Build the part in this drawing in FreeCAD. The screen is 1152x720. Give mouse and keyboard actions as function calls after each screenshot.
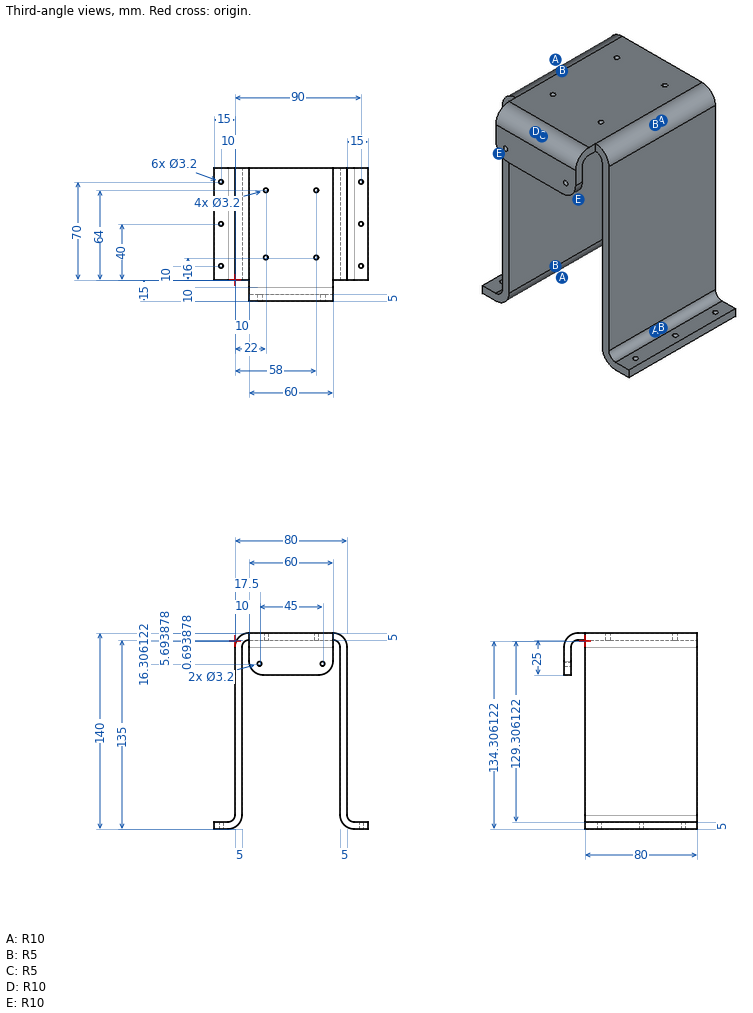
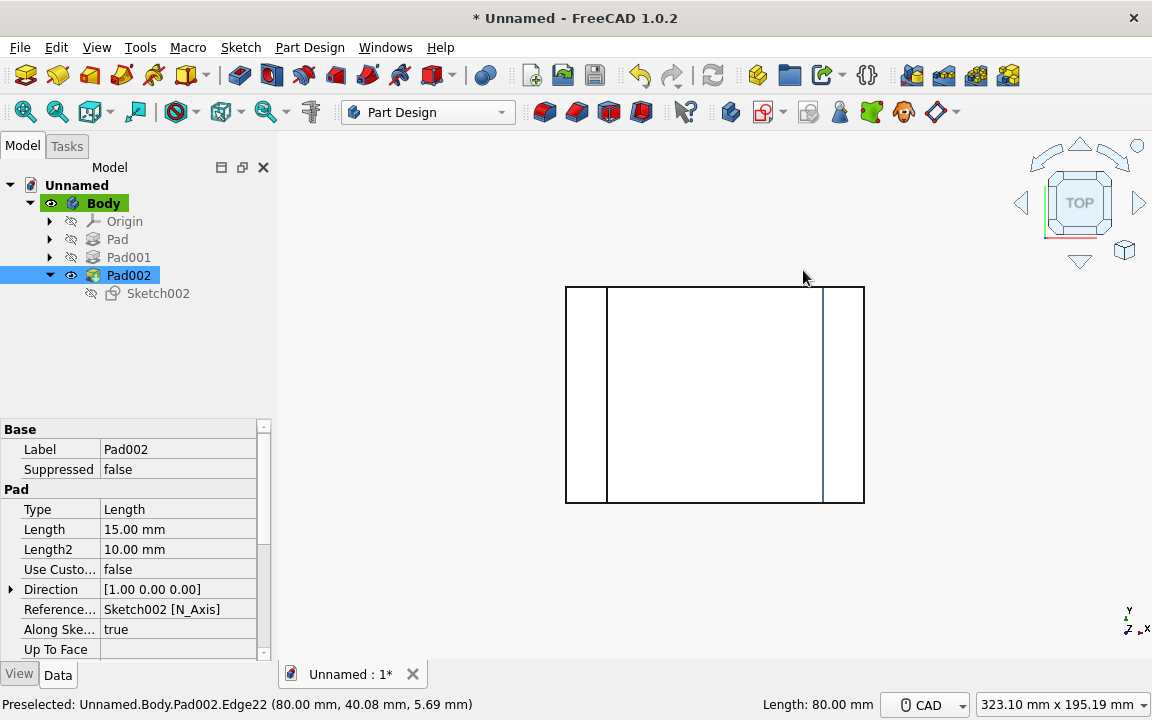
click(26, 112)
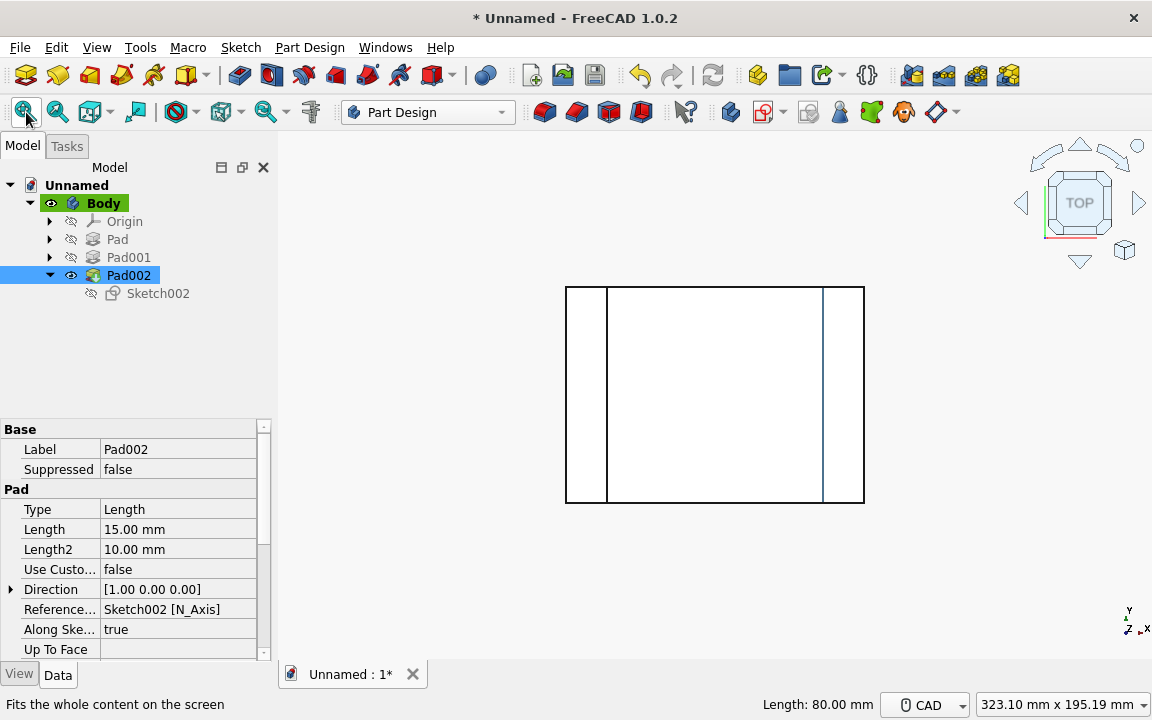
click(607, 394, ctrl)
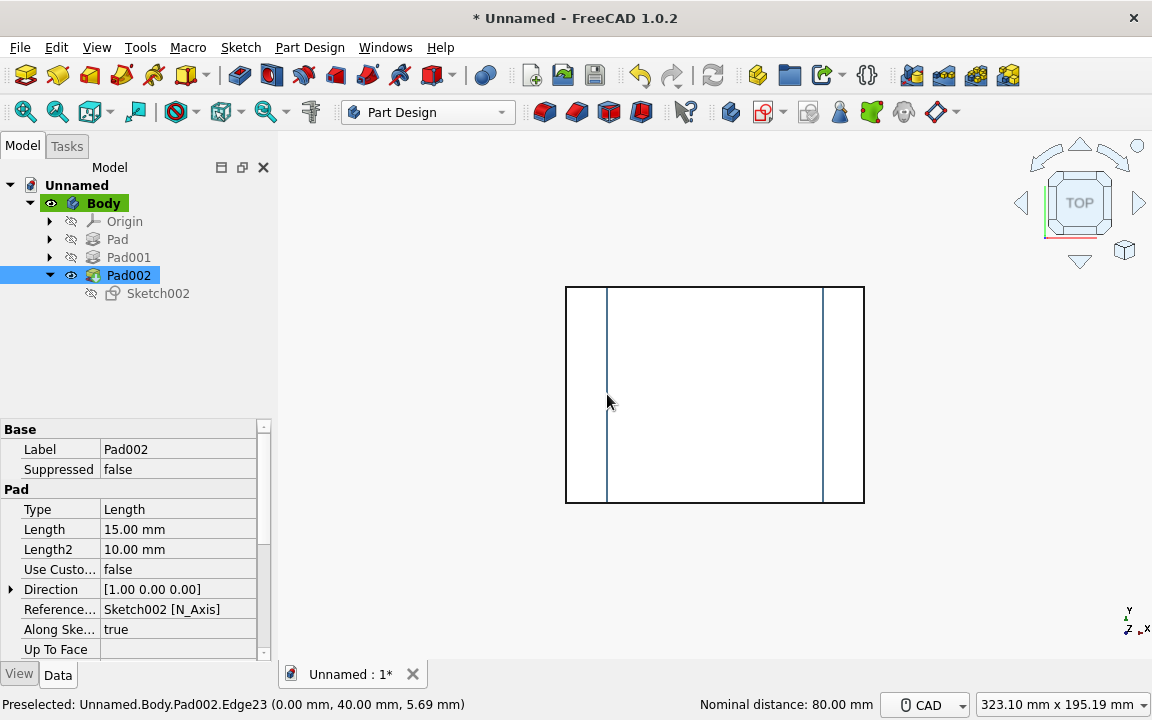
key(1)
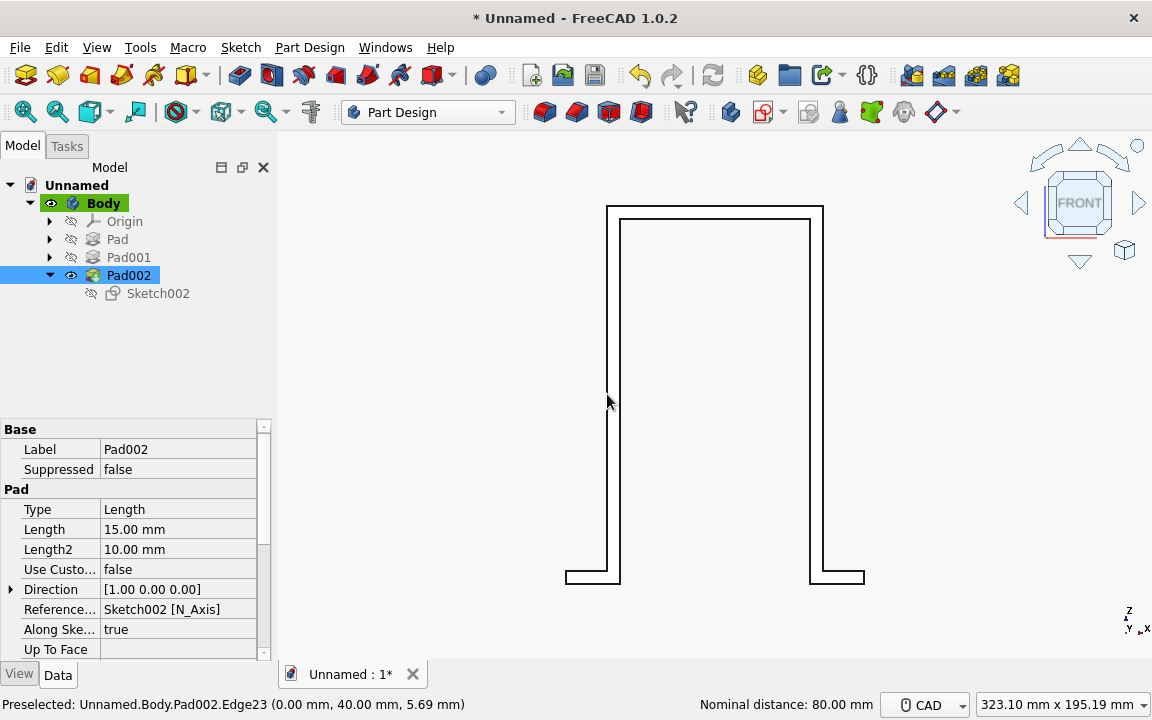
key(3)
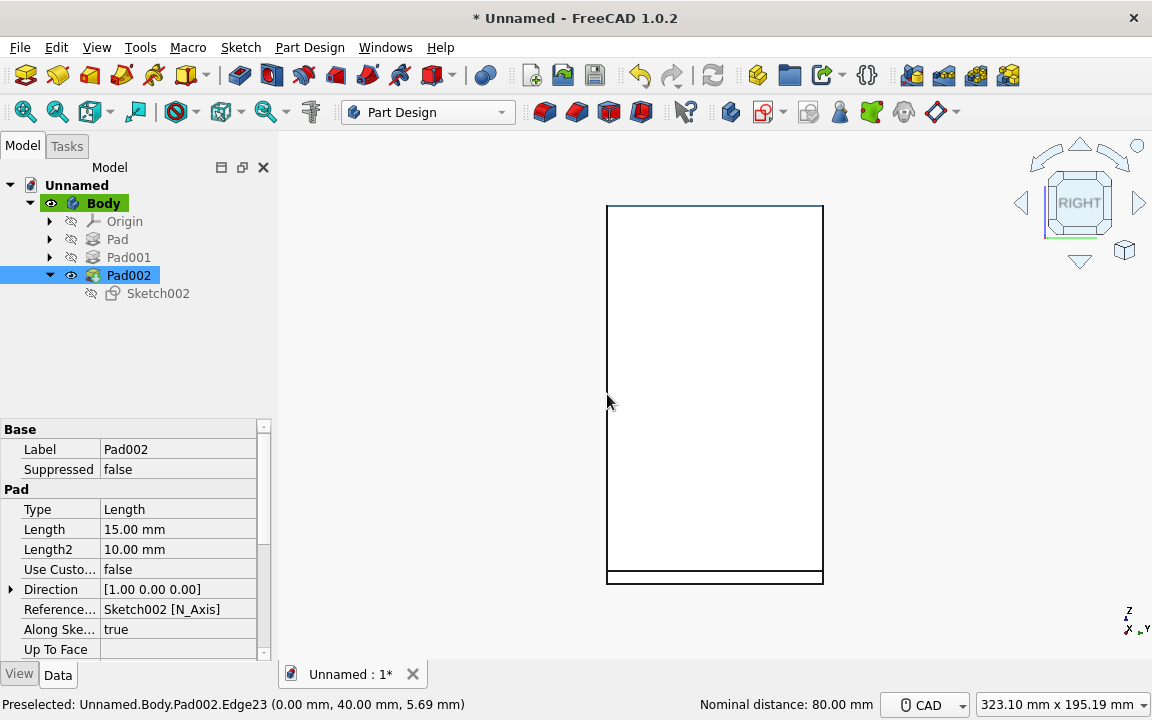
key(5)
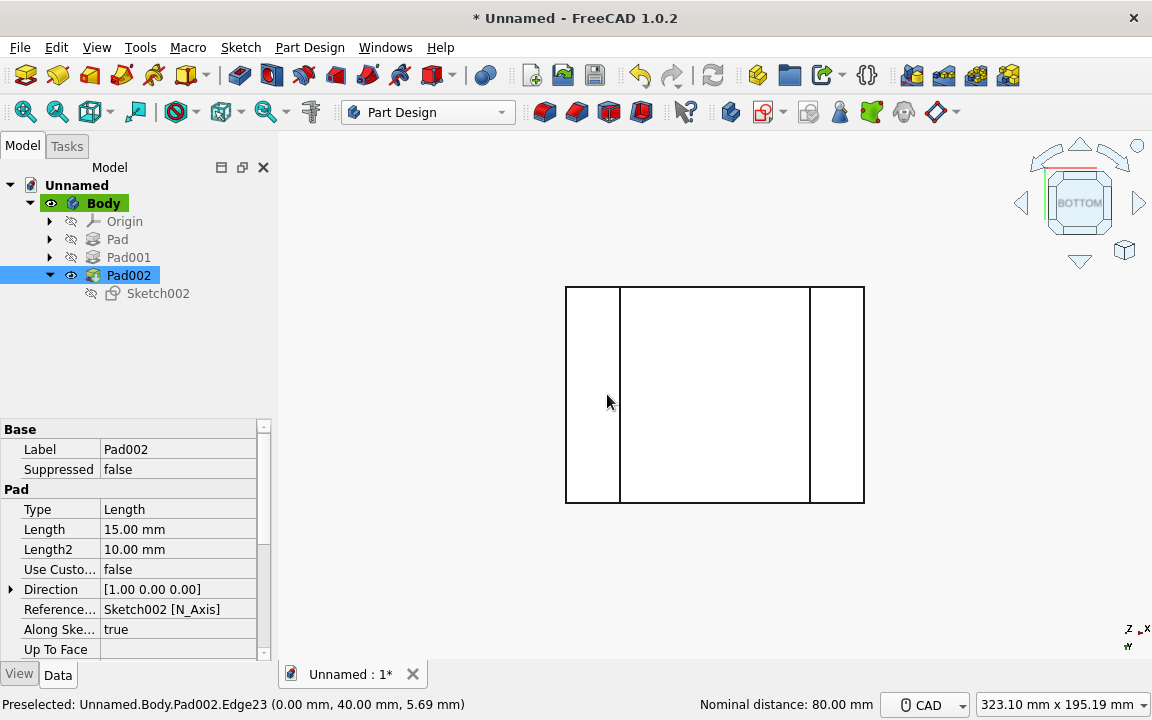
click(26, 112)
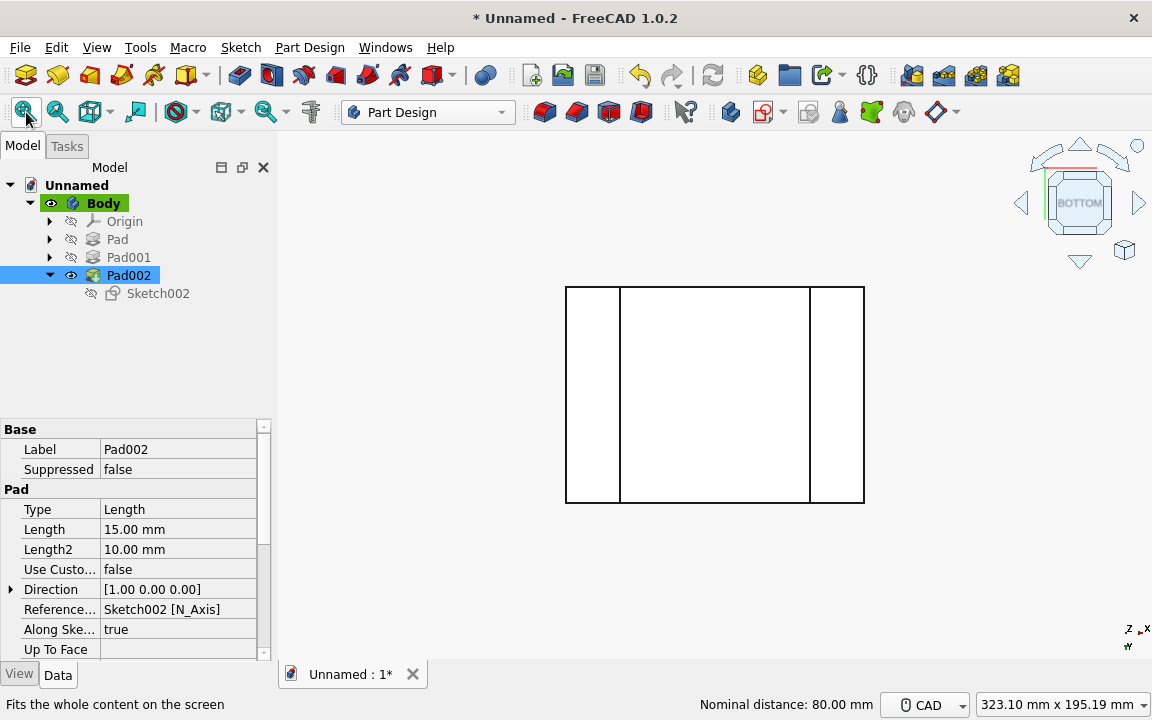
click(620, 394, ctrl)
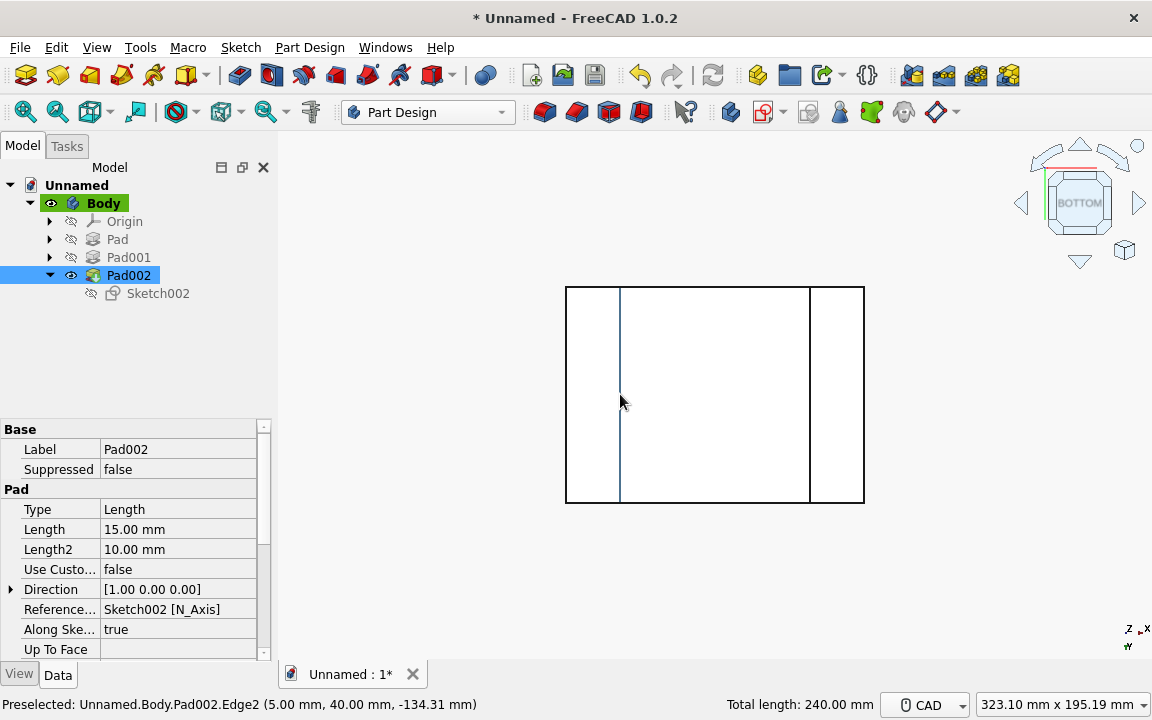
click(810, 394, ctrl)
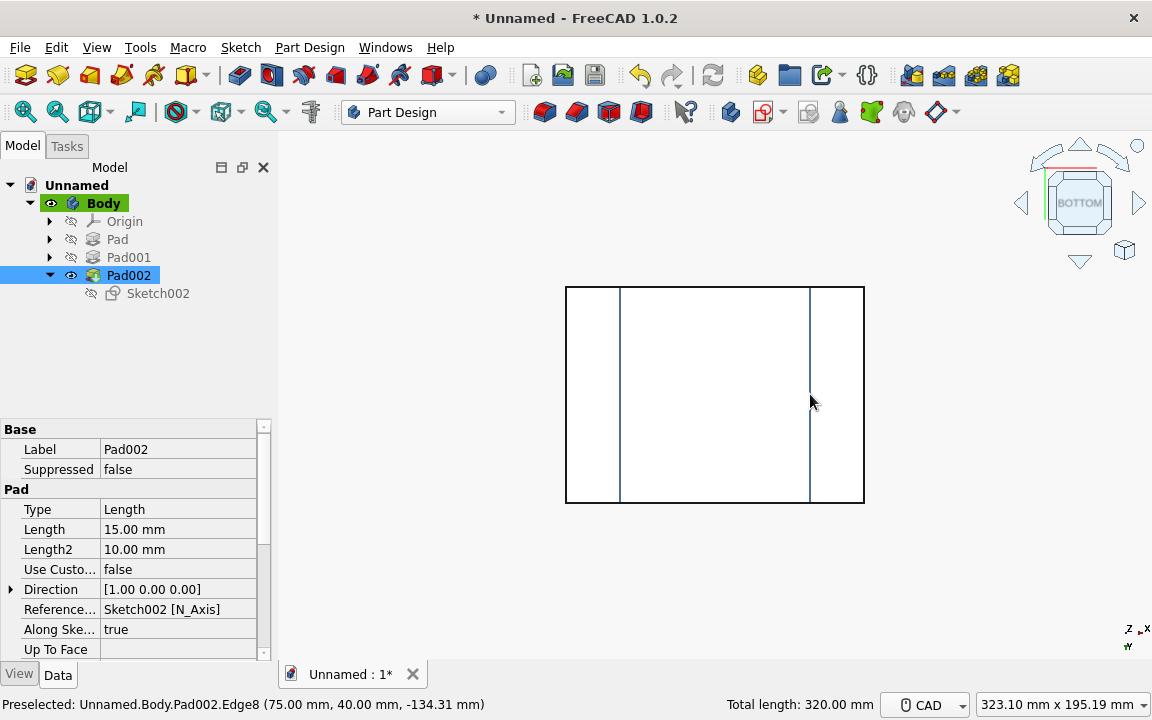
click(546, 112)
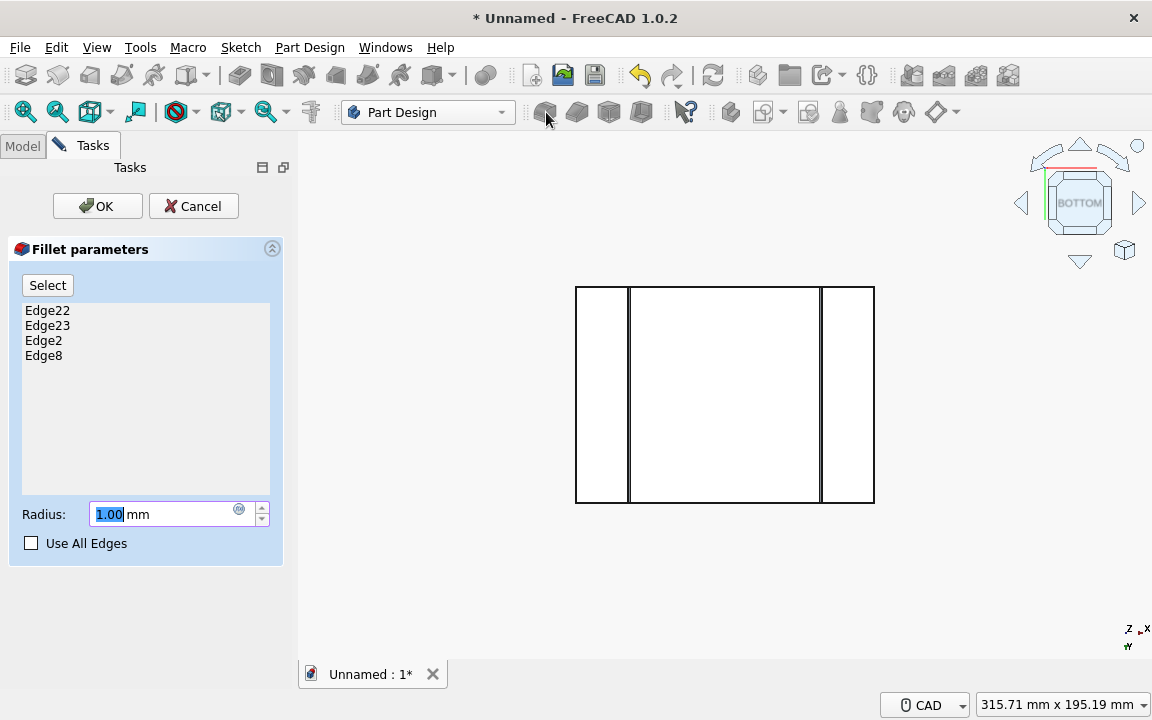
text(10)
key(Tab)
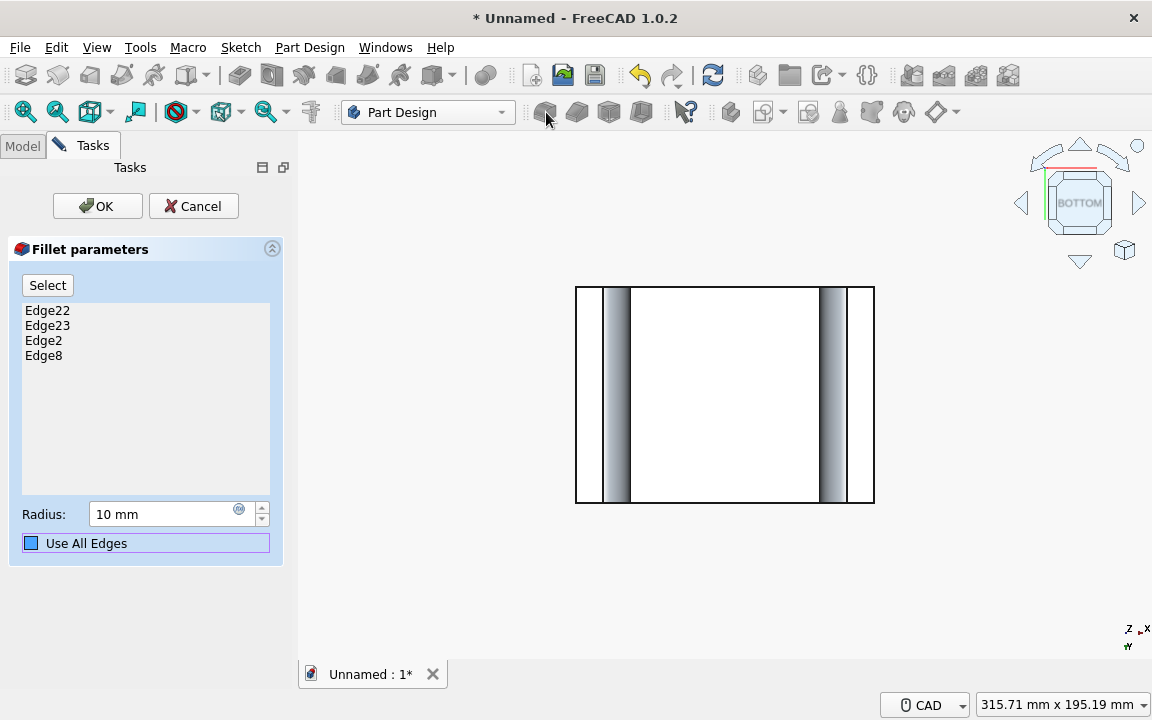
click(98, 206)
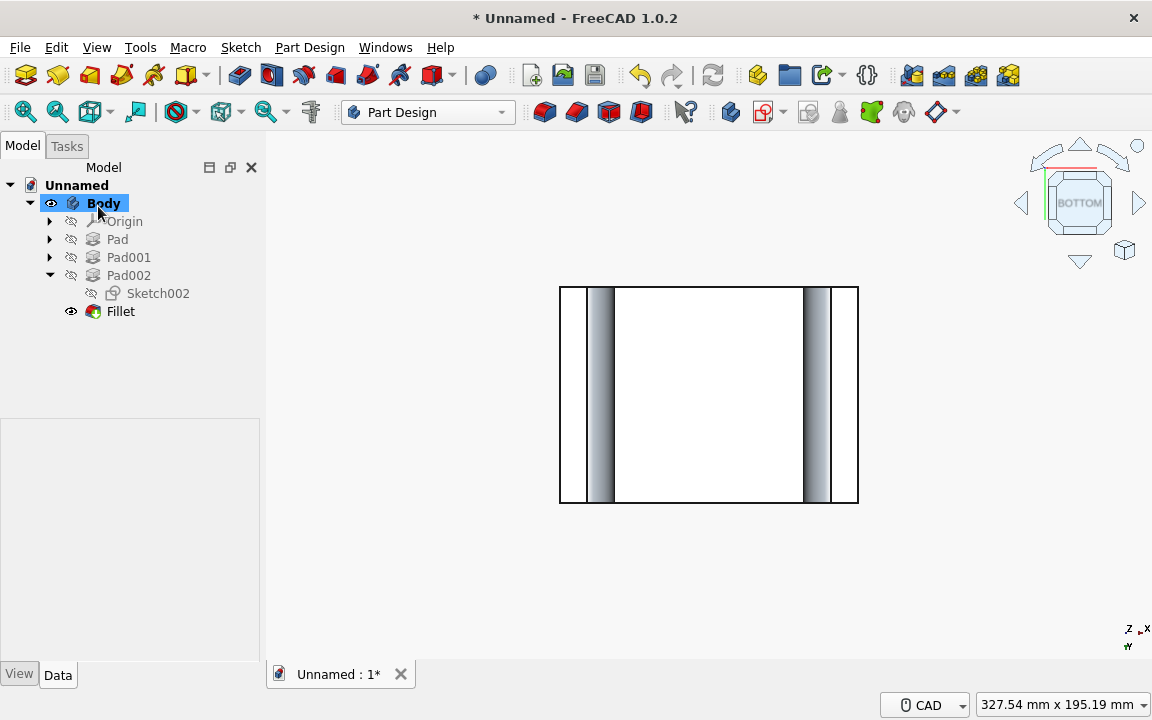
click(26, 112)